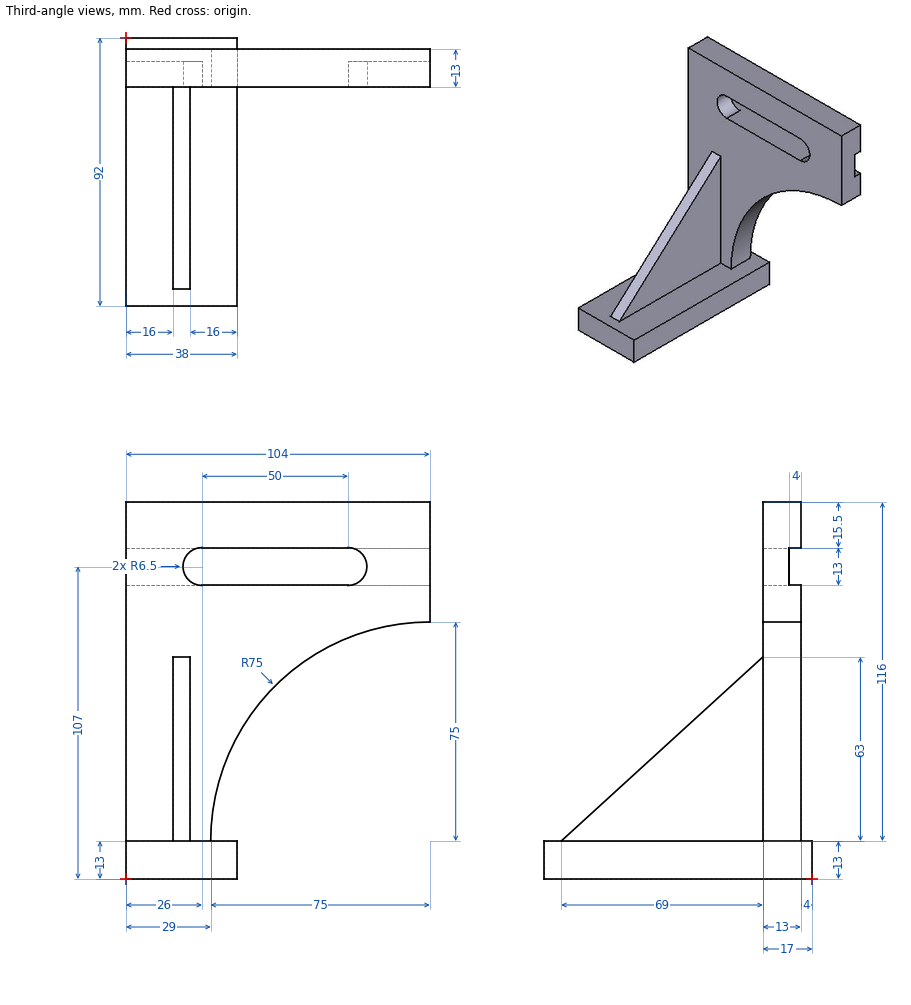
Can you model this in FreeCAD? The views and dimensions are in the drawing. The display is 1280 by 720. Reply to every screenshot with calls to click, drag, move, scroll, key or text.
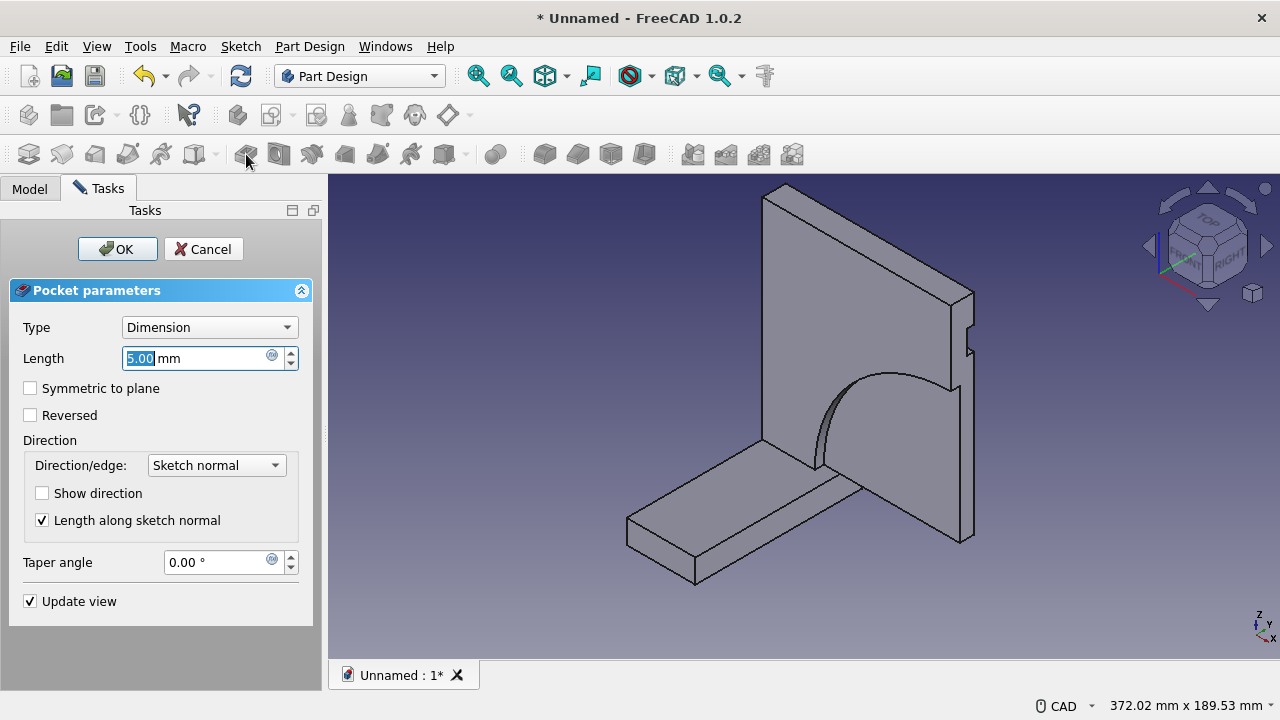
text(13)
key(Tab)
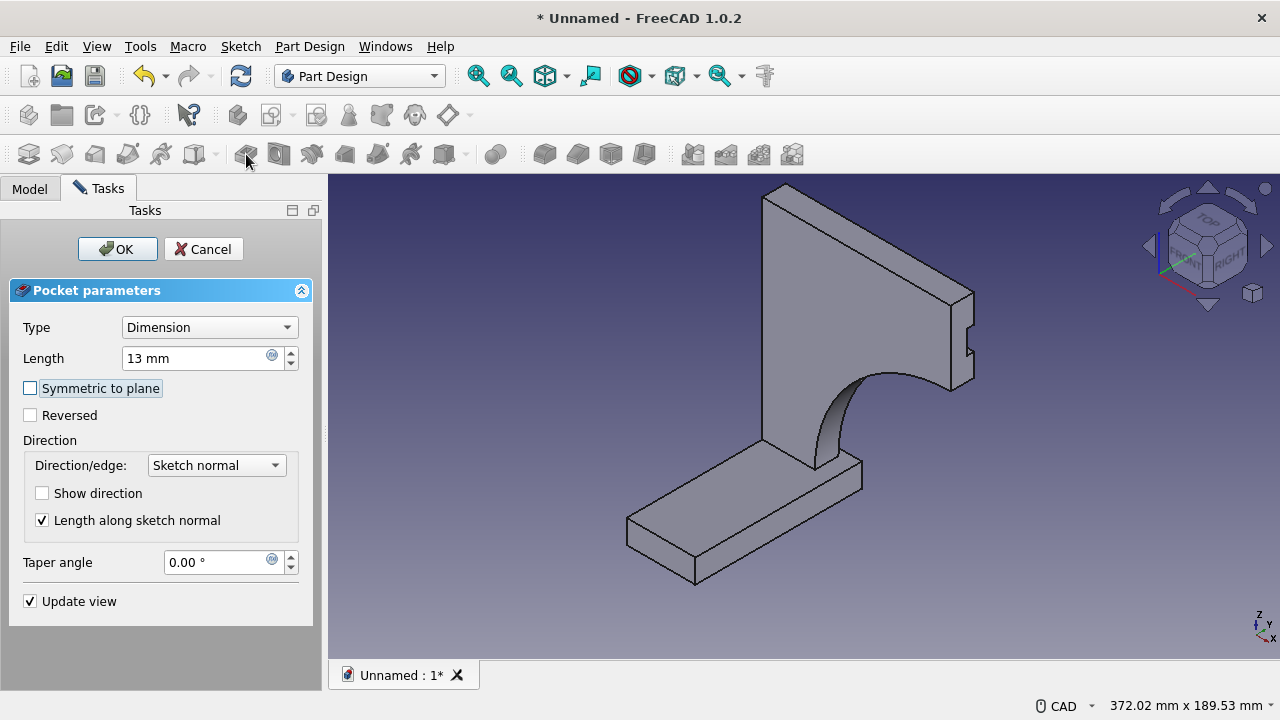
click(118, 249)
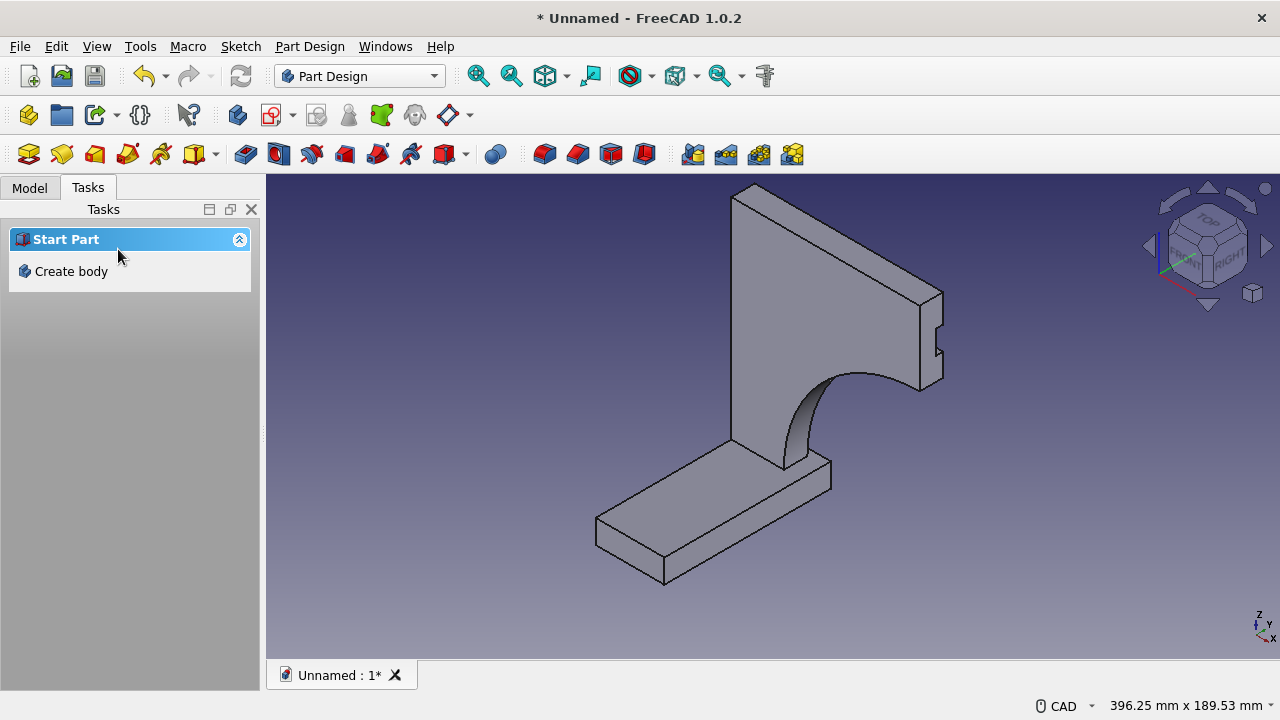
click(799, 321)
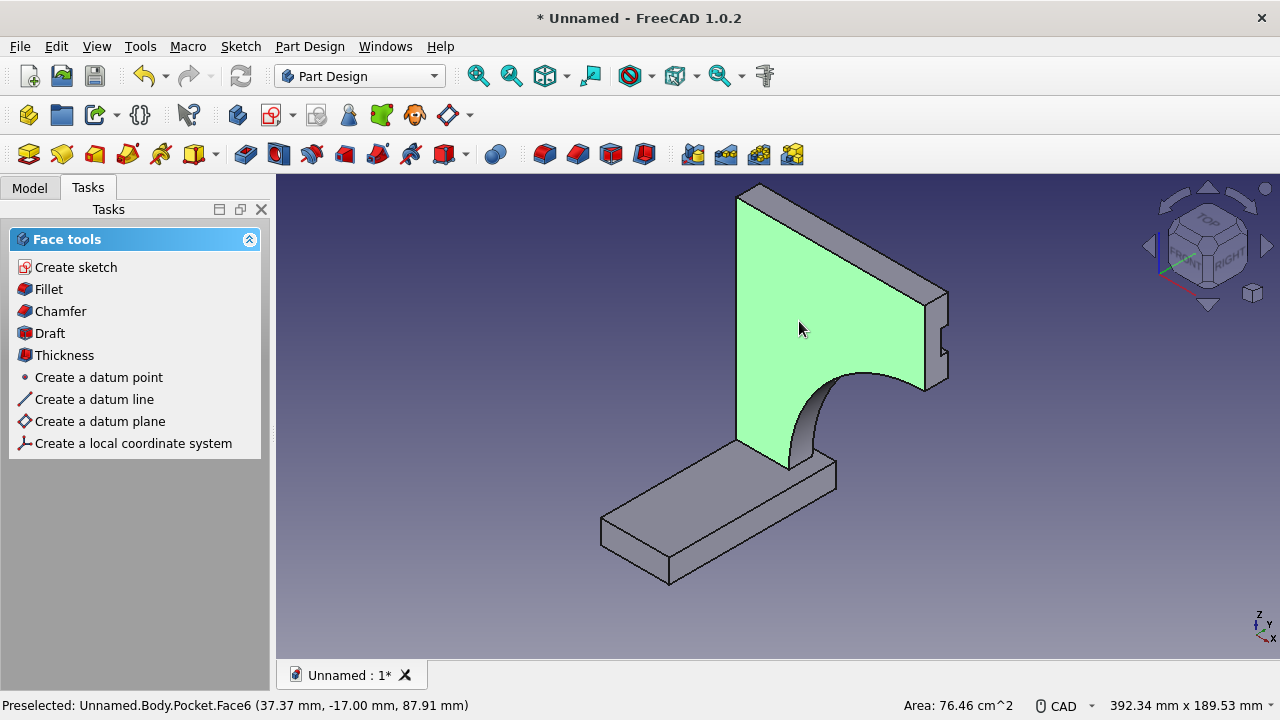
click(270, 116)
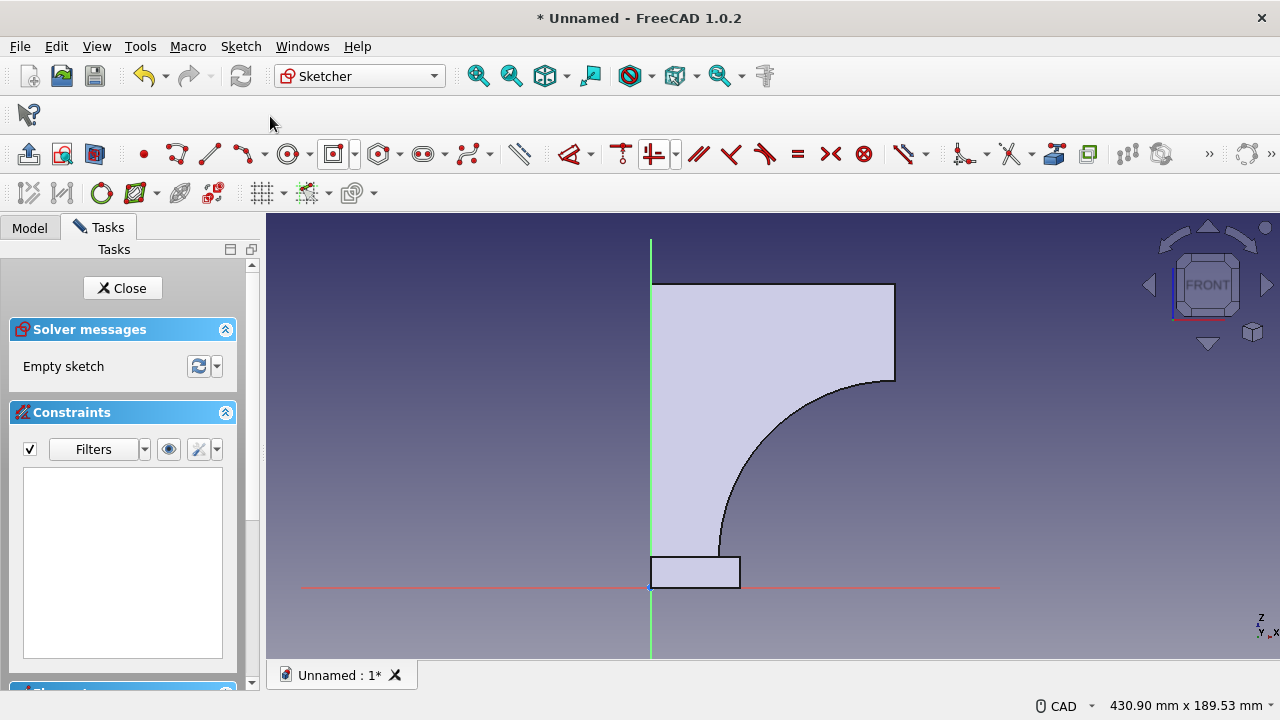
key(q)
key(s)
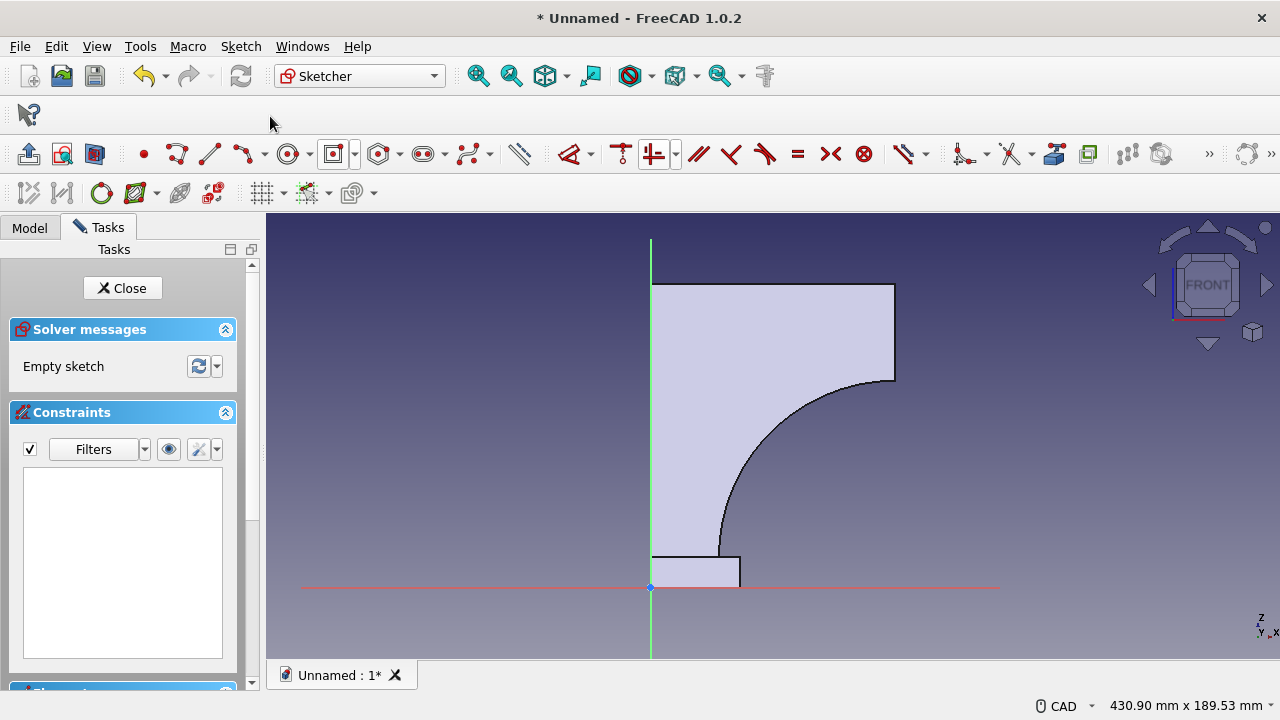
click(422, 154)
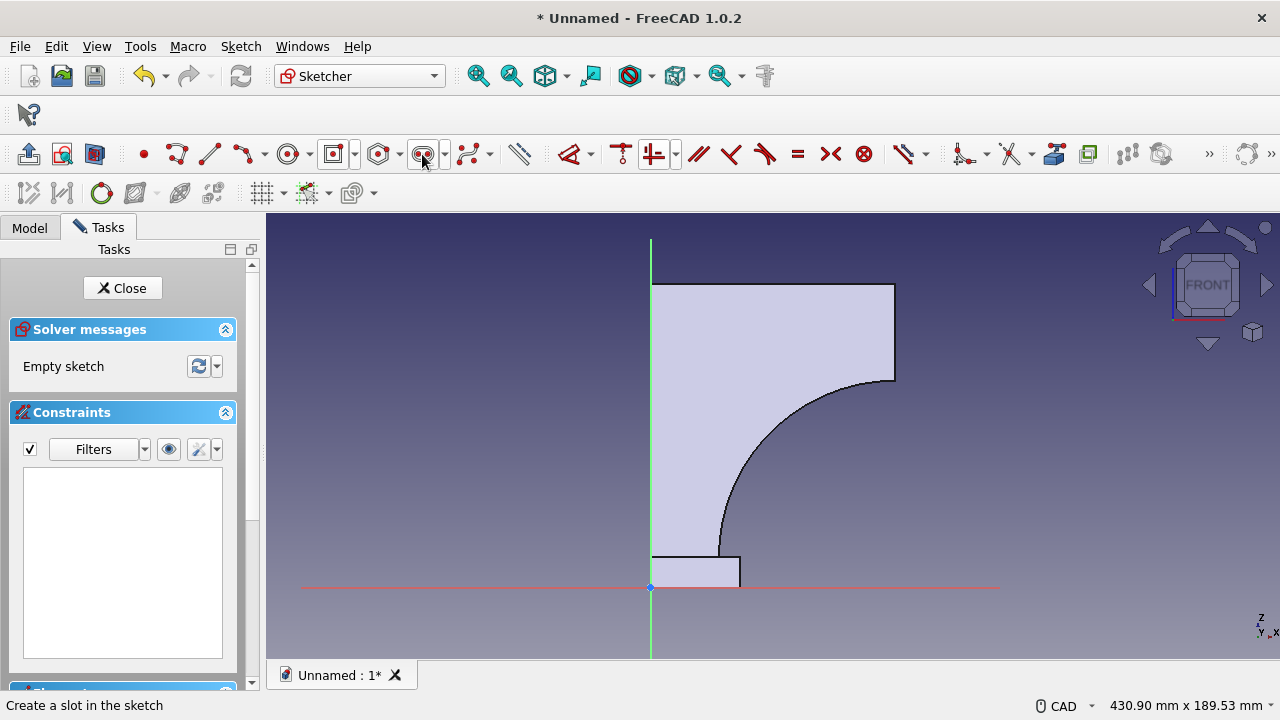
scroll(712, 336, up, 2)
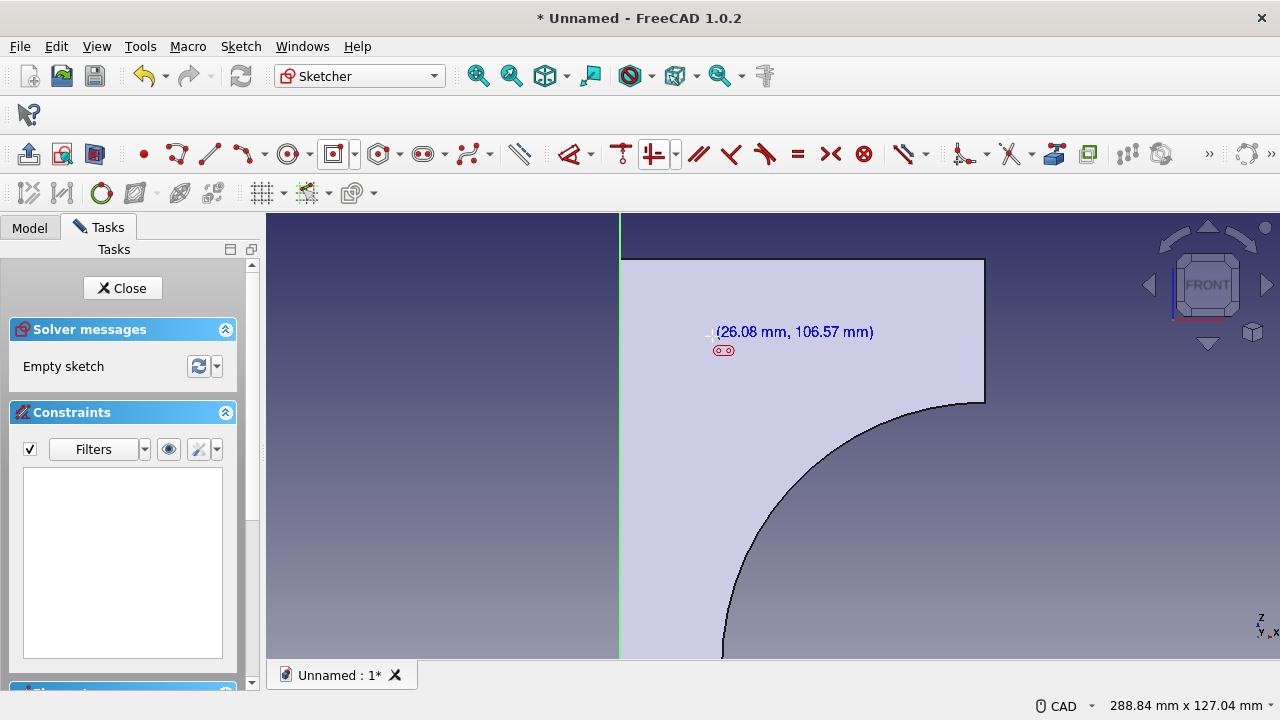
click(712, 336)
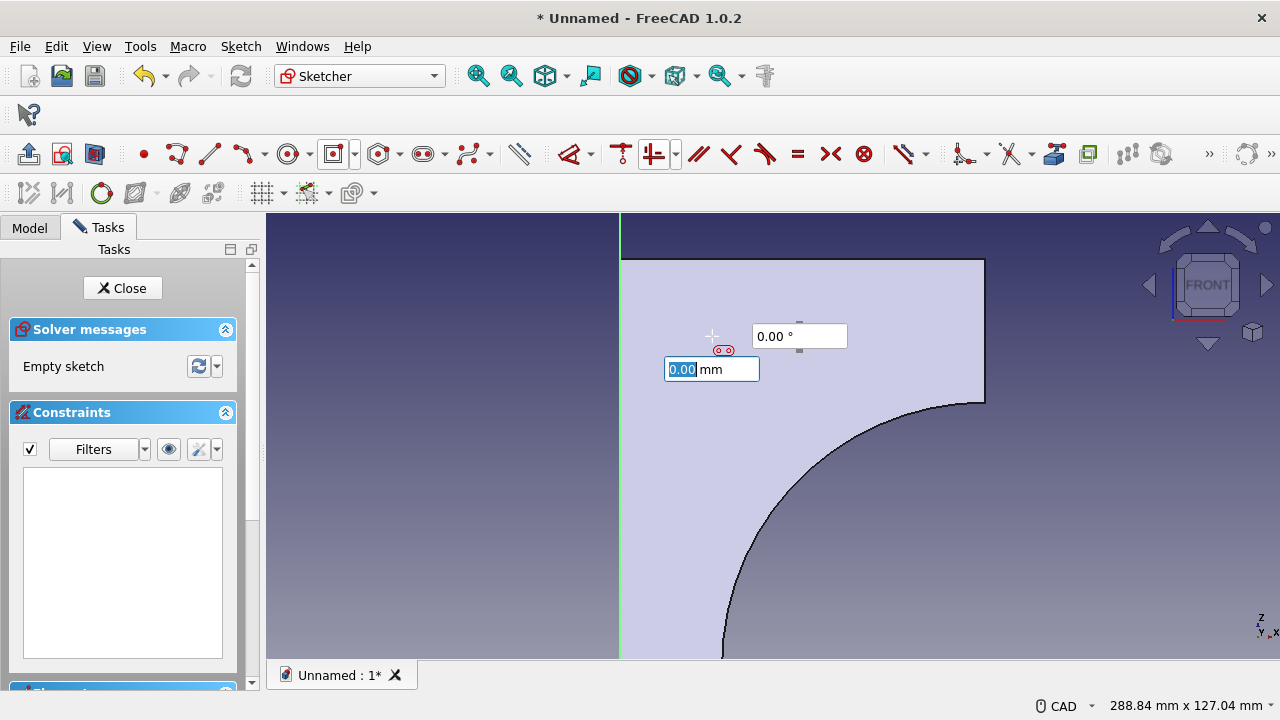
click(887, 336)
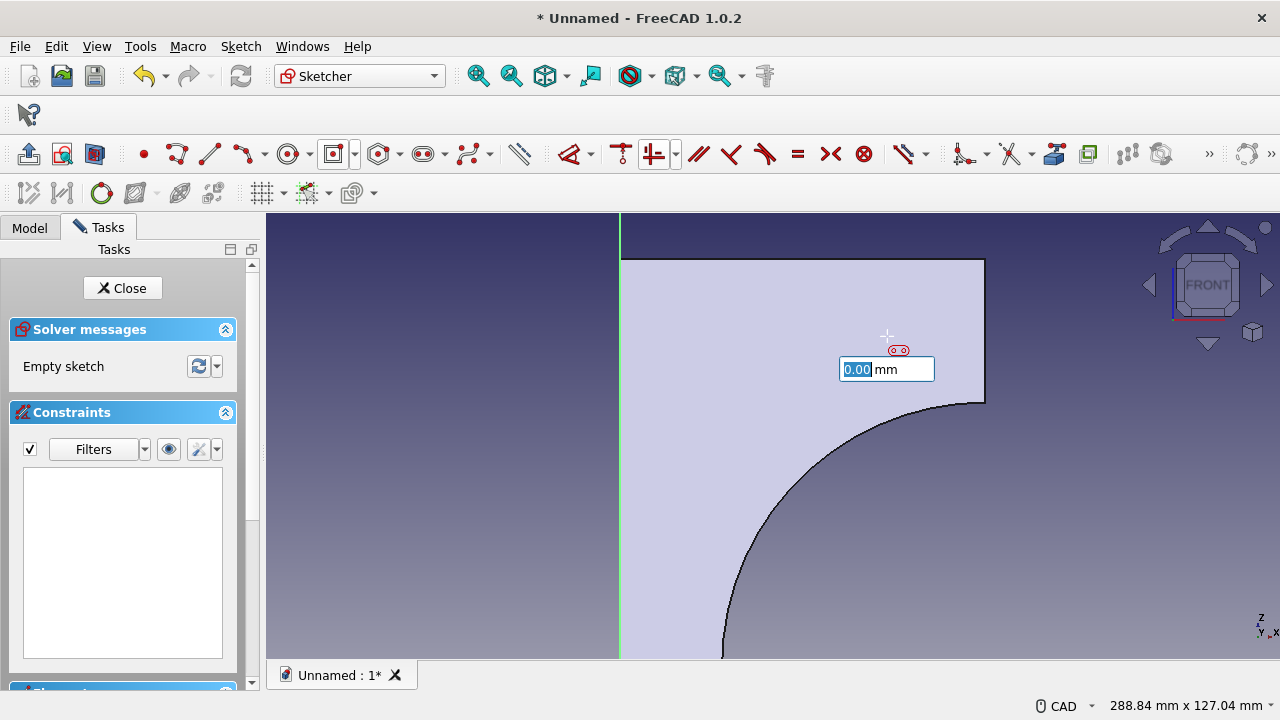
click(799, 313)
key(Escape)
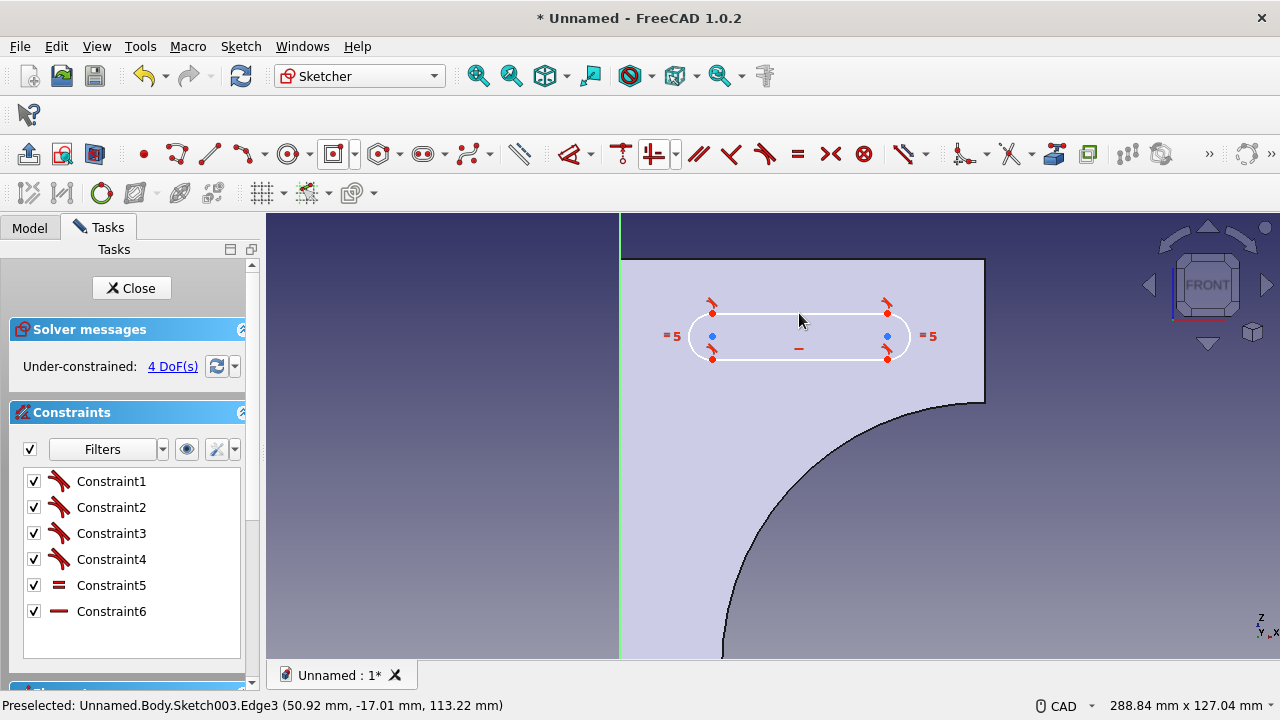
click(568, 154)